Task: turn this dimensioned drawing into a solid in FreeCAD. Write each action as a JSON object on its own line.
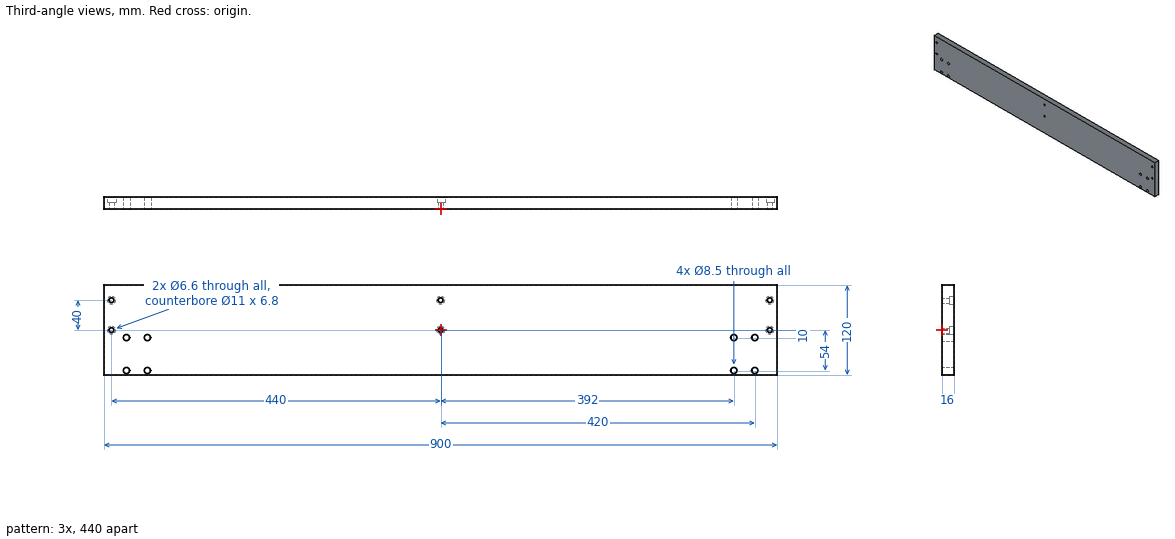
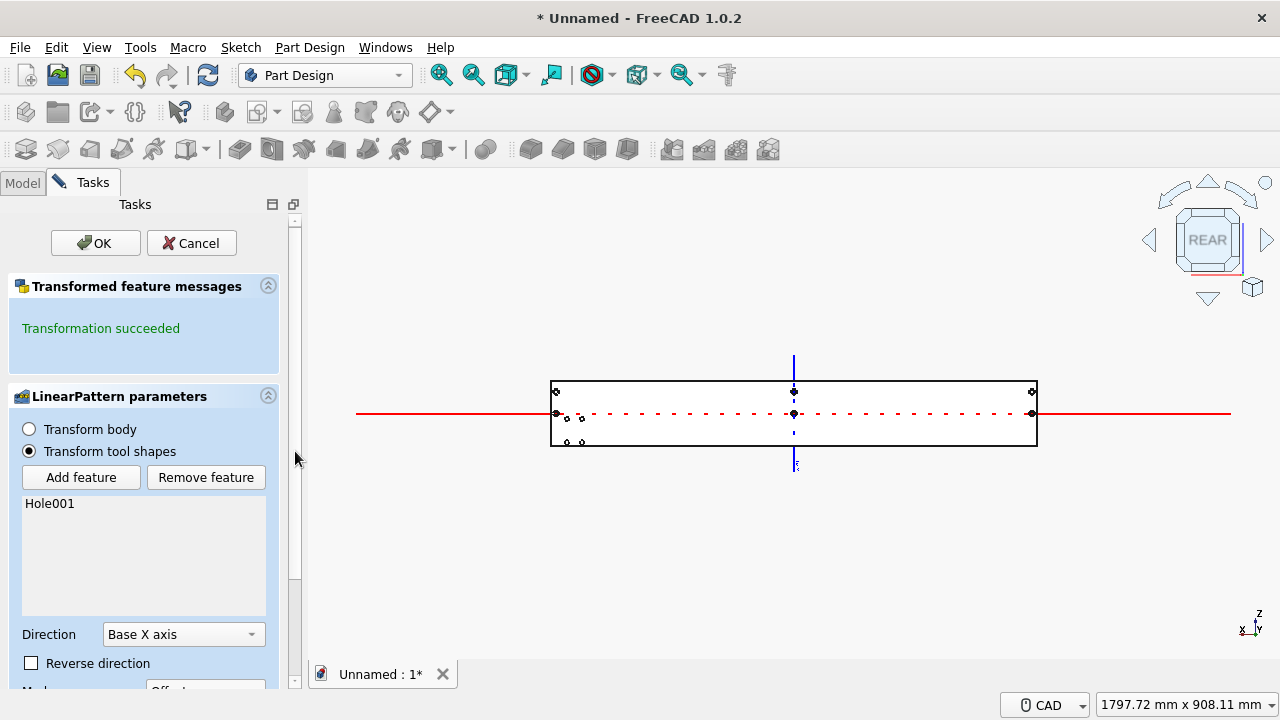
{"action": "left_click", "coordinate": [96, 243]}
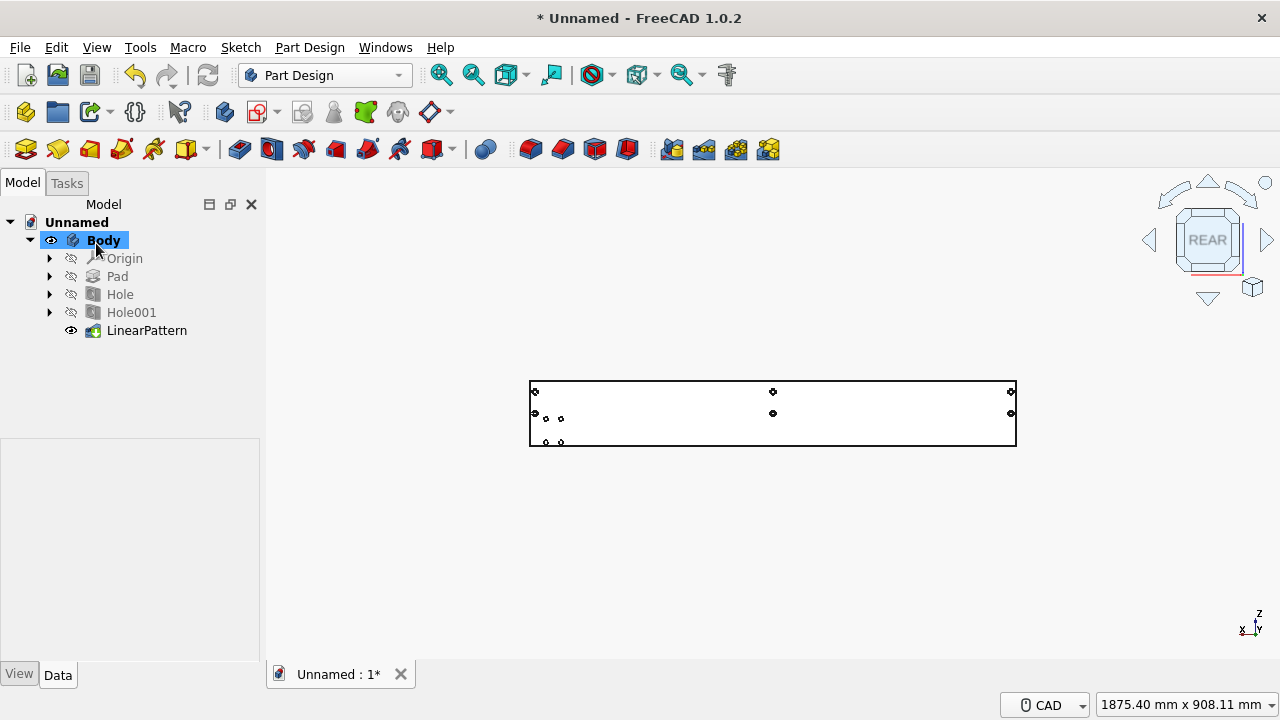
{"action": "left_click", "coordinate": [116, 294]}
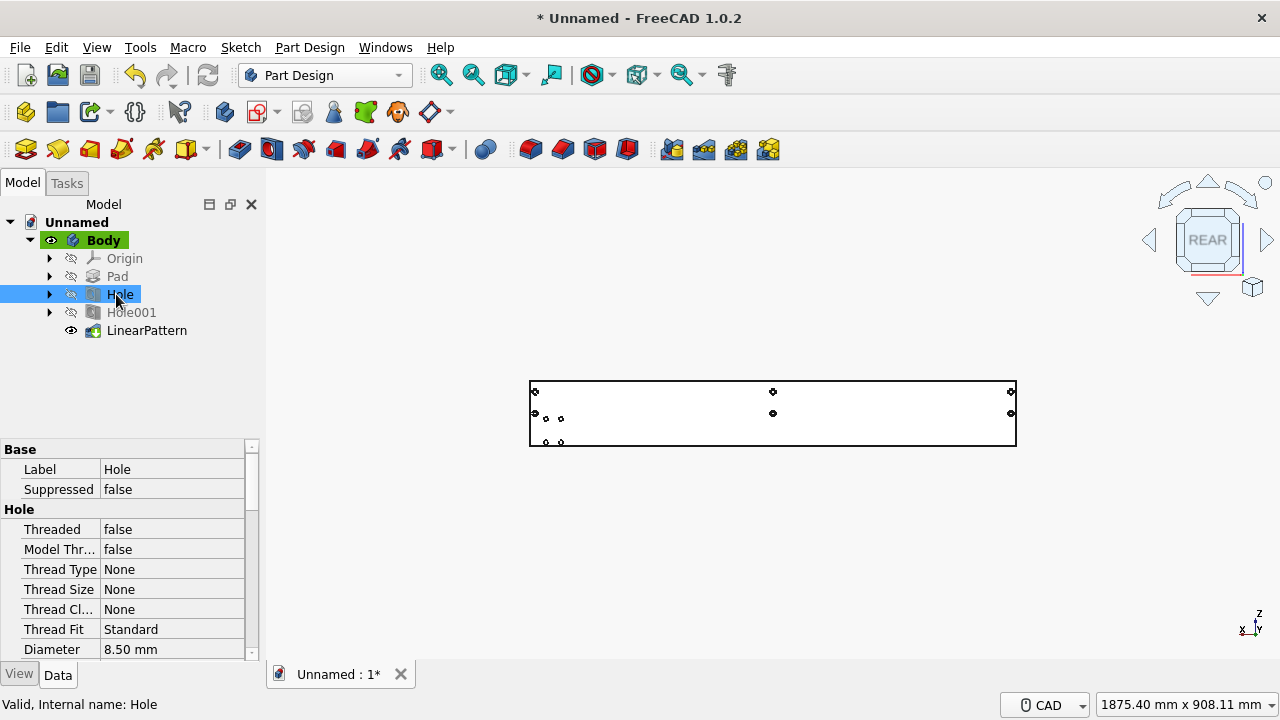
{"action": "left_click", "coordinate": [672, 150]}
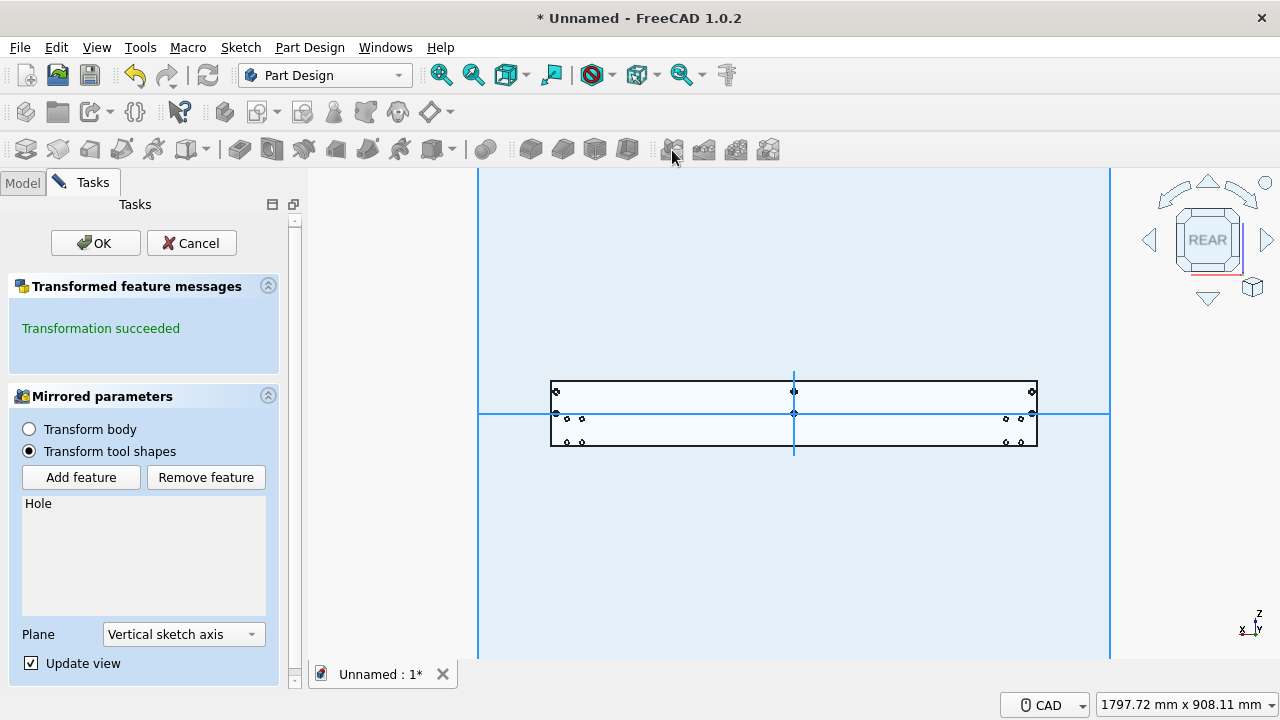
{"action": "left_click", "coordinate": [184, 634]}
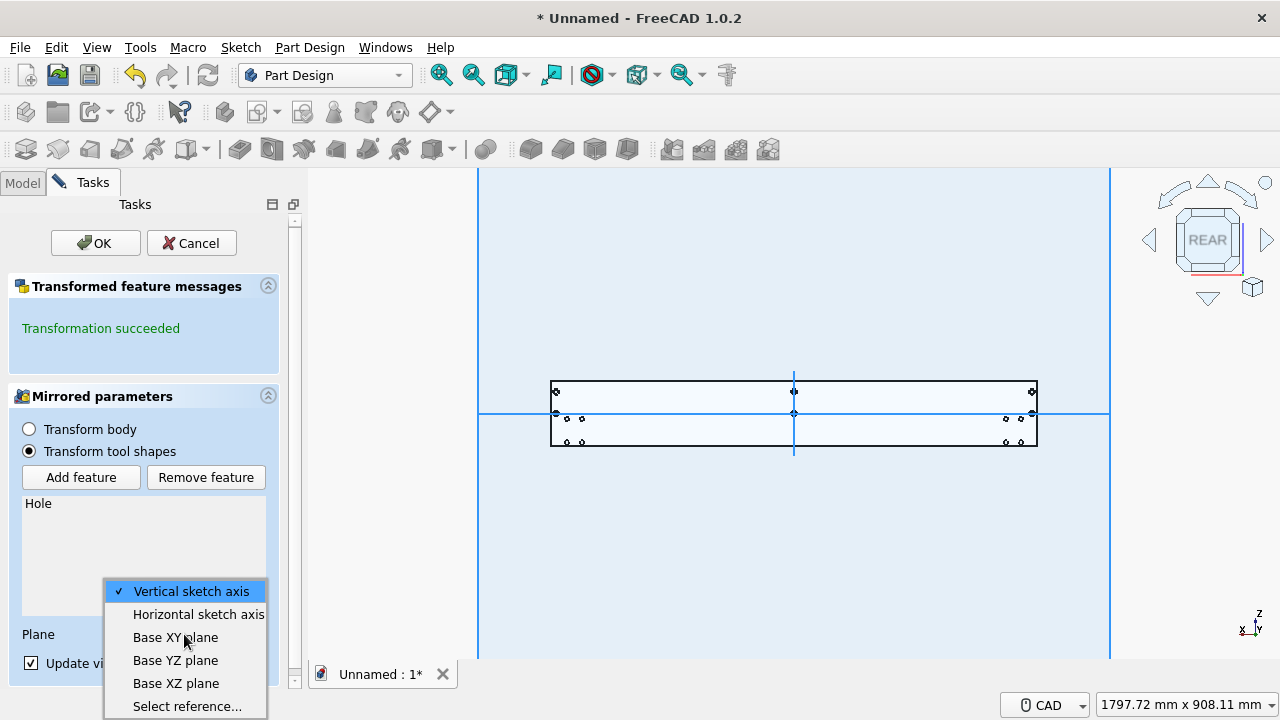
{"action": "left_click", "coordinate": [184, 660]}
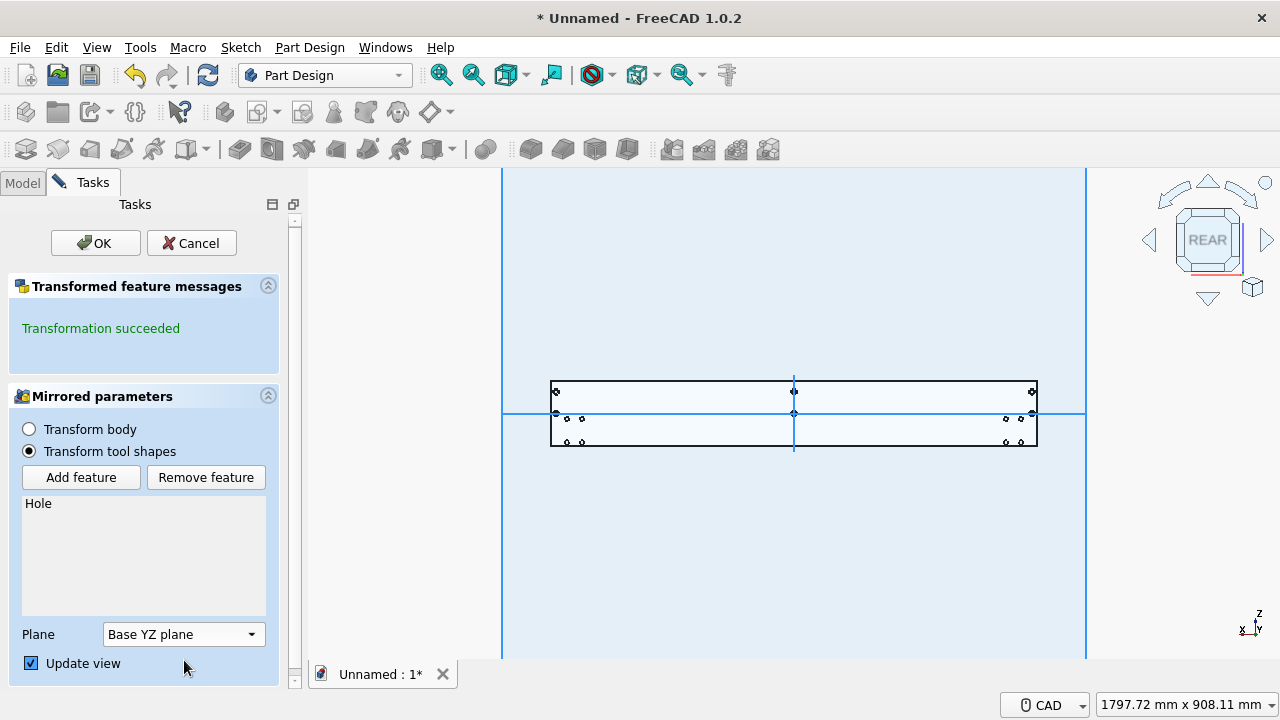
{"action": "left_click", "coordinate": [96, 243]}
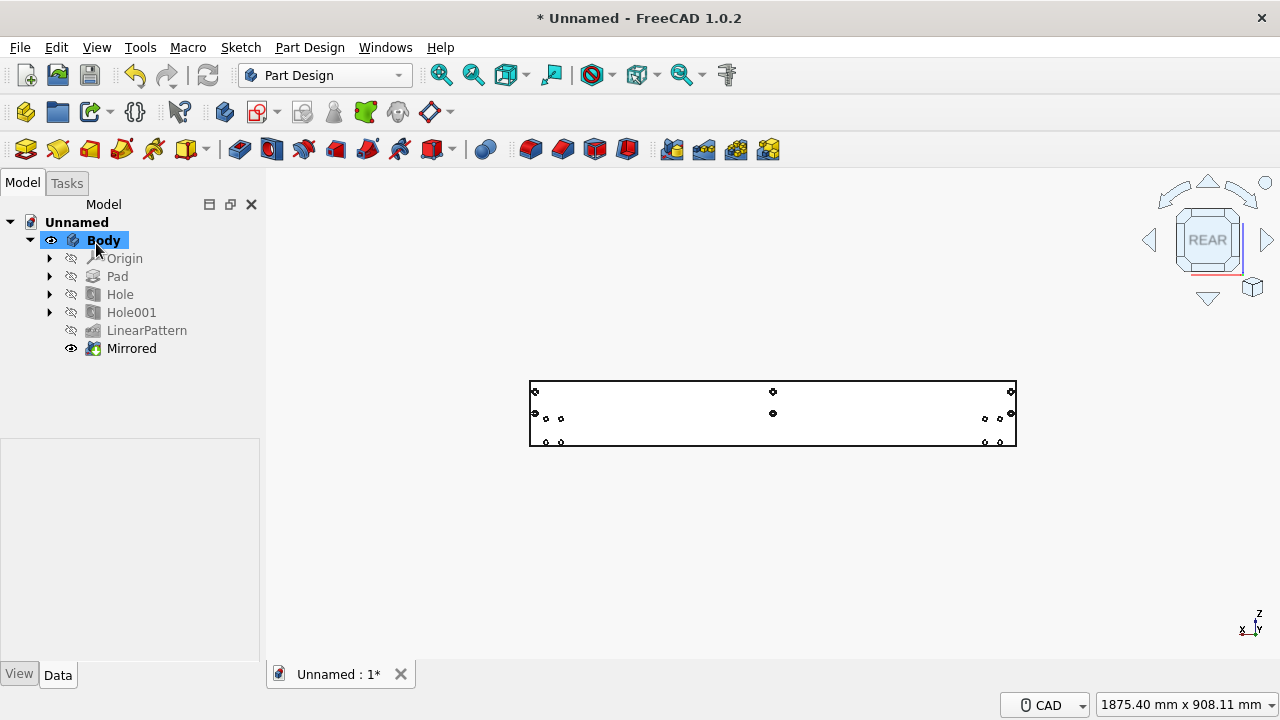
{"action": "key", "text": "0"}